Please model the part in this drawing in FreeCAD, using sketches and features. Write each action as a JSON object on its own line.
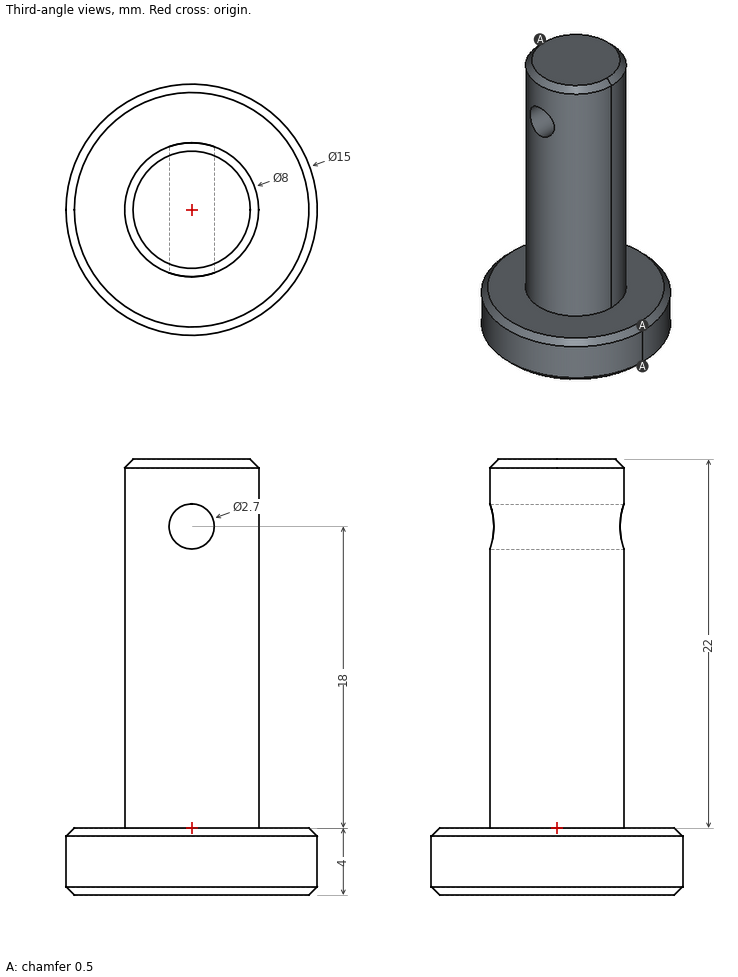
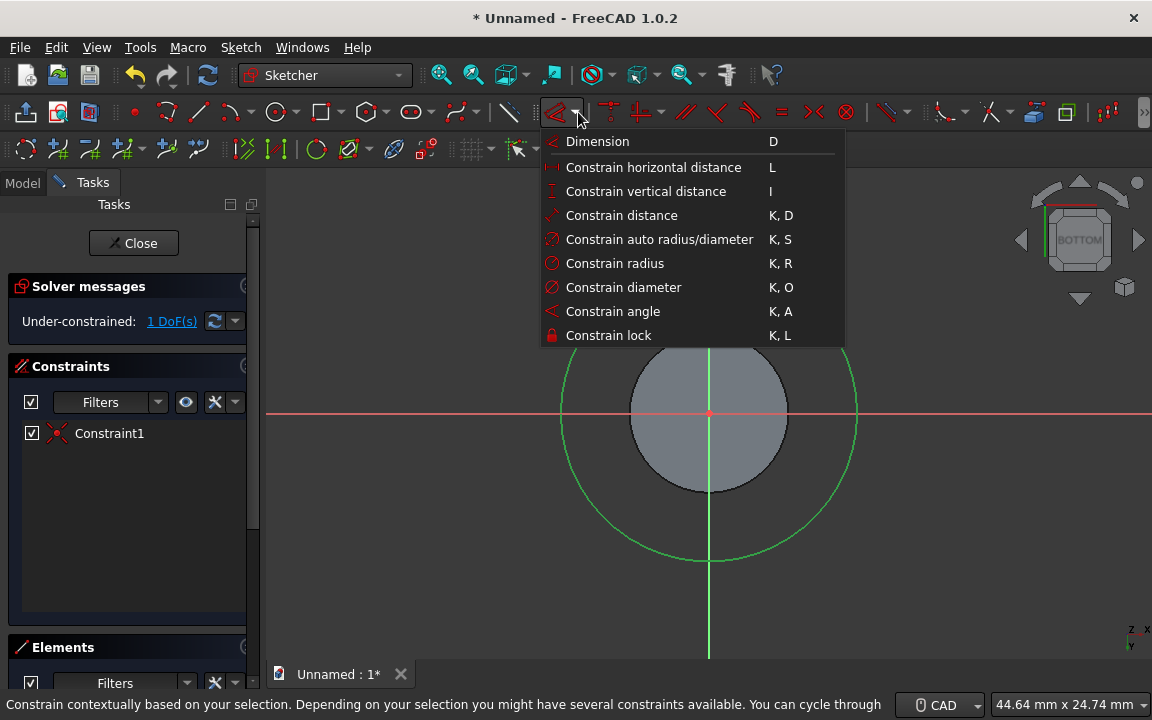
{"action": "left_click", "coordinate": [693, 287]}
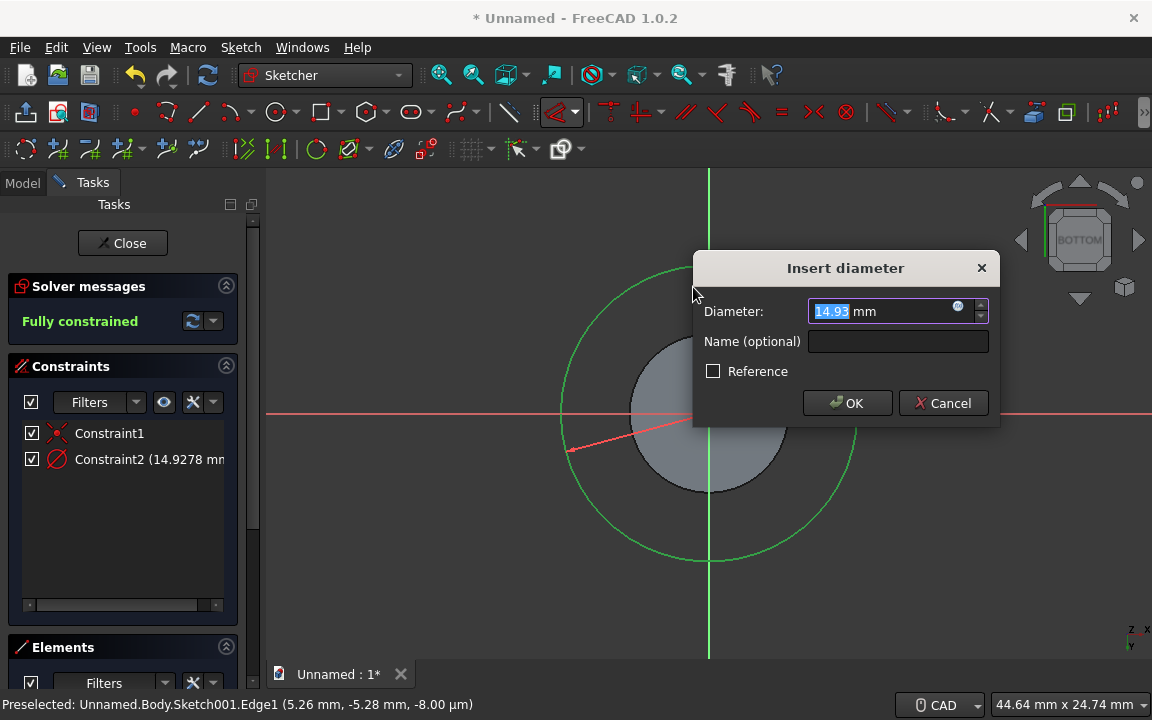
{"action": "type", "text": "15"}
{"action": "key", "text": "Return"}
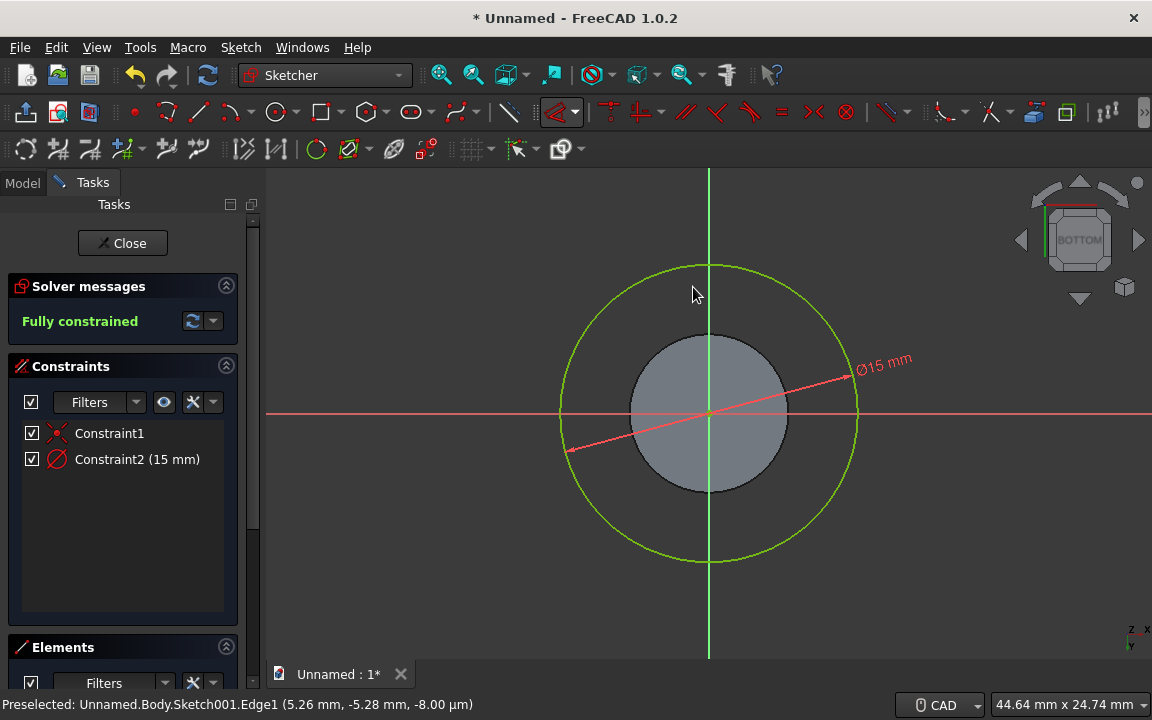
{"action": "left_click", "coordinate": [123, 243]}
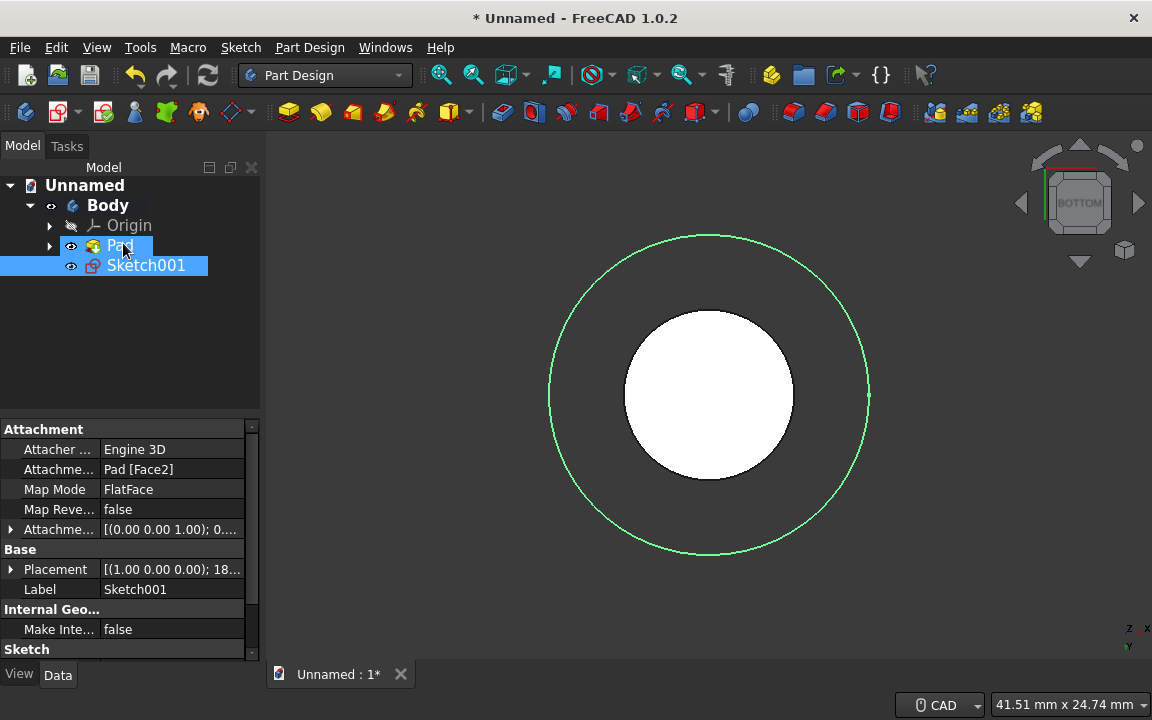
{"action": "left_click", "coordinate": [290, 112]}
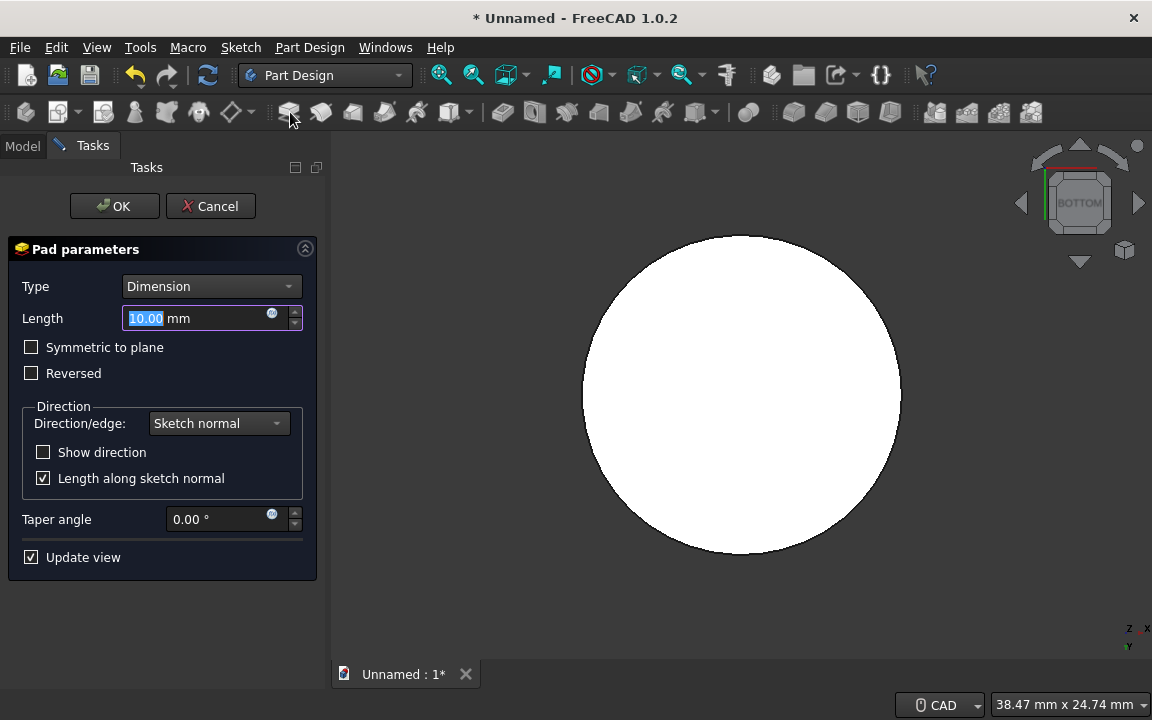
{"action": "type", "text": "4"}
{"action": "key", "text": "Tab"}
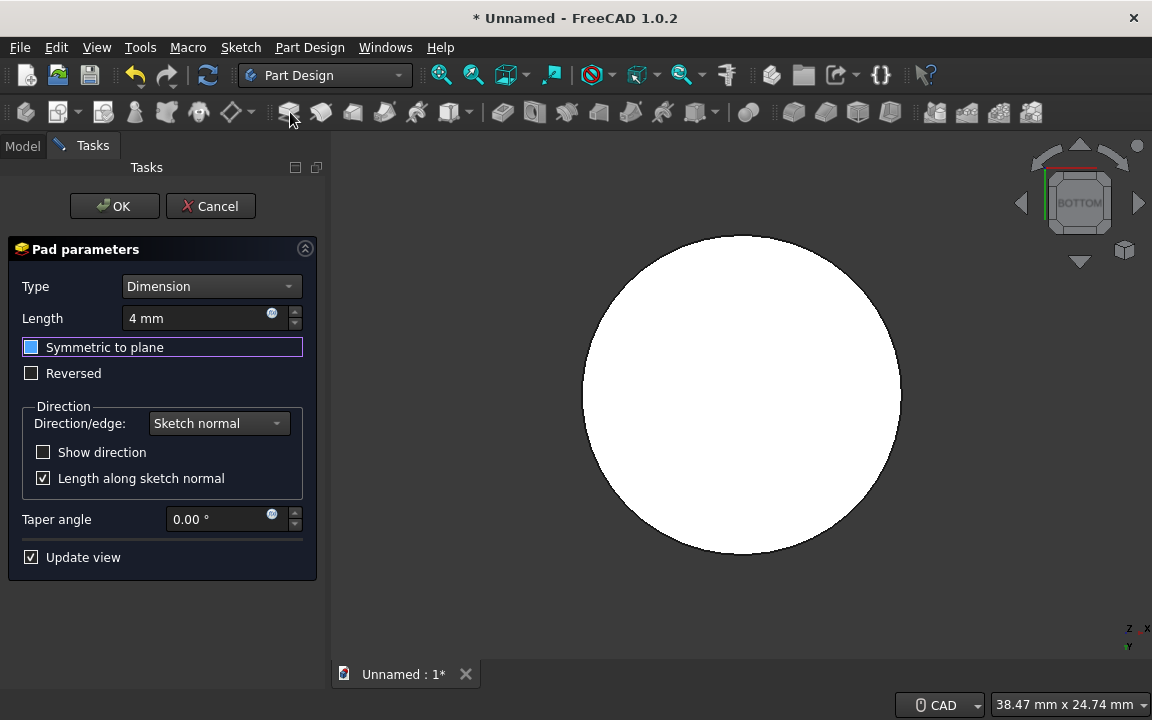
{"action": "left_click", "coordinate": [115, 206]}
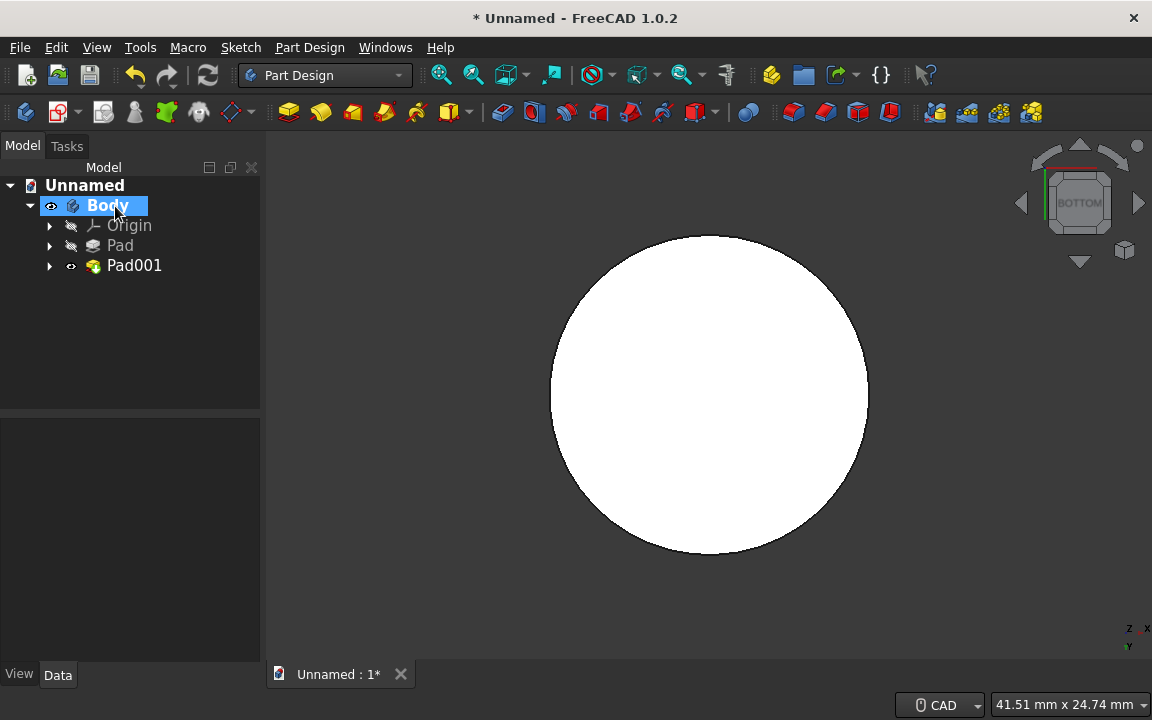
{"action": "left_click", "coordinate": [58, 112]}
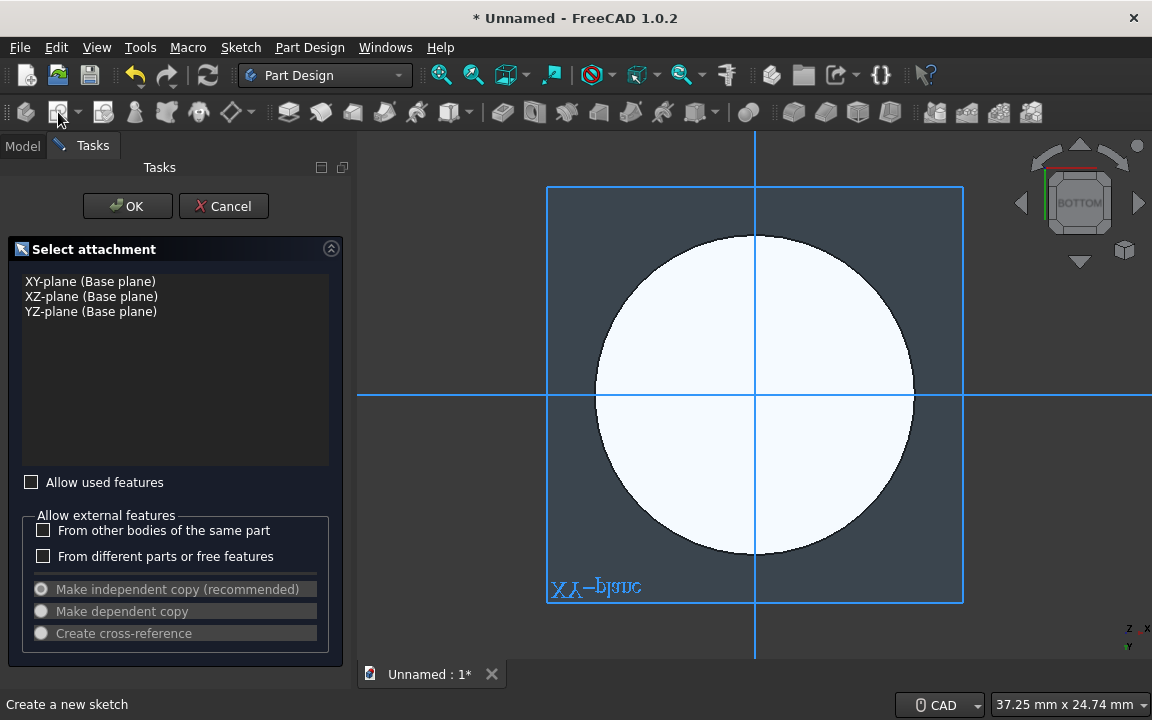
{"action": "left_click", "coordinate": [82, 296]}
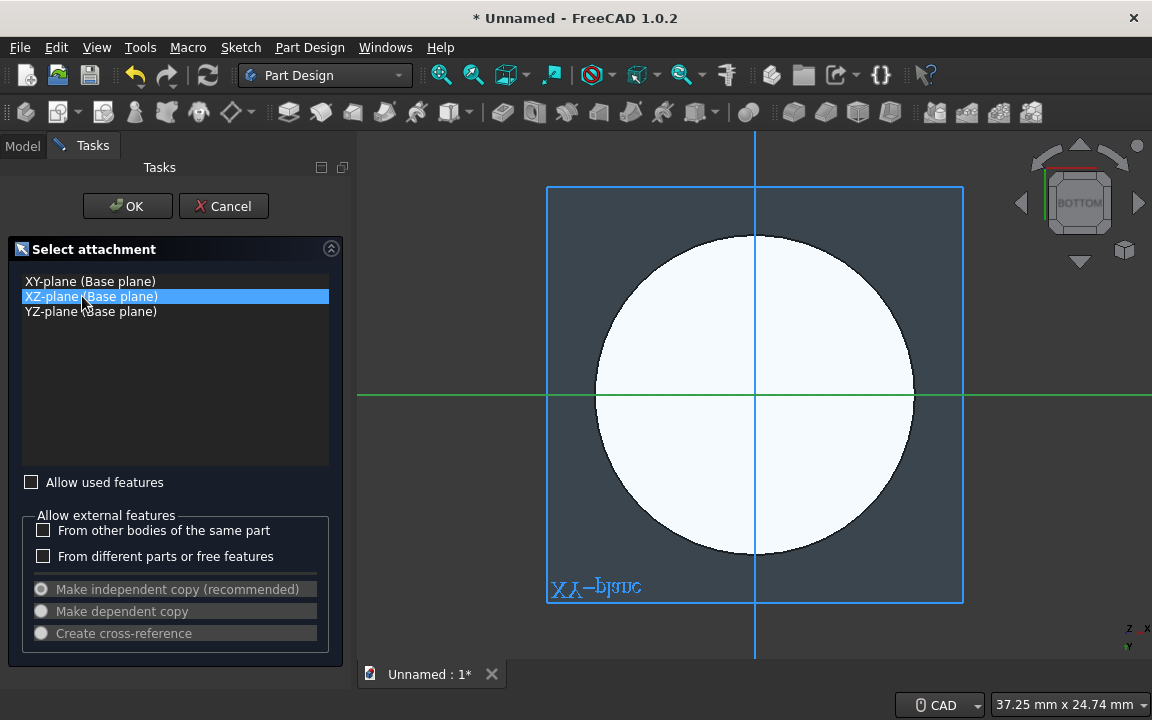
{"action": "left_click", "coordinate": [128, 206]}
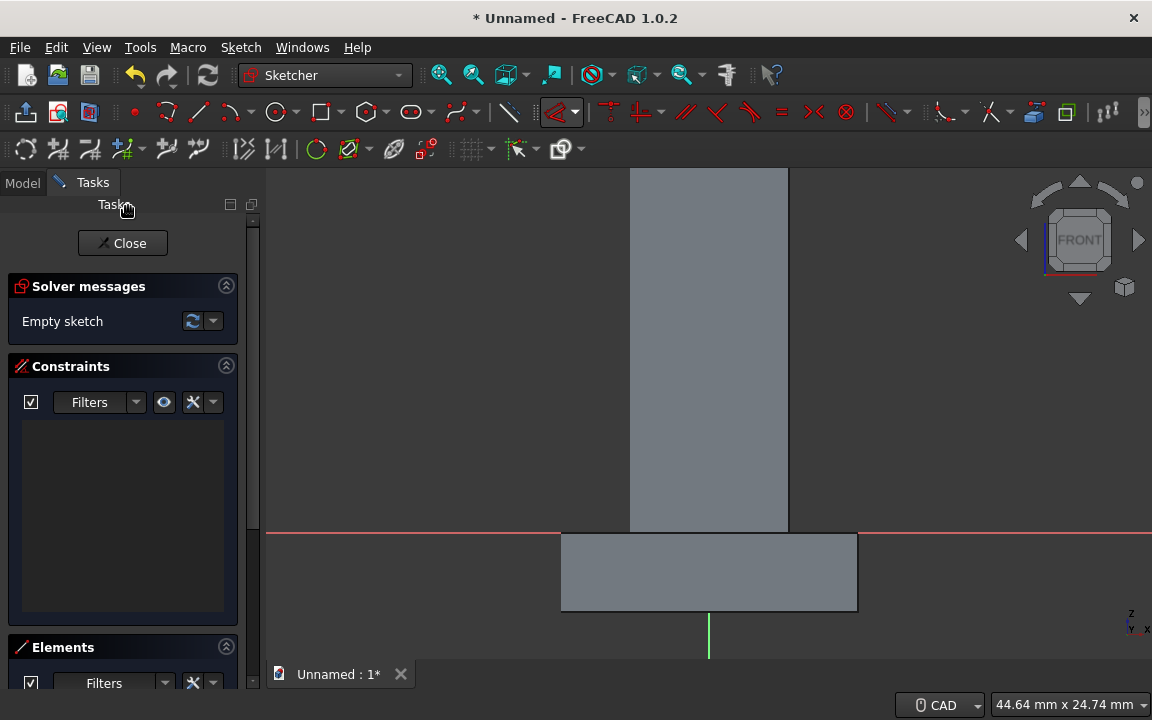
{"action": "left_click", "coordinate": [90, 112]}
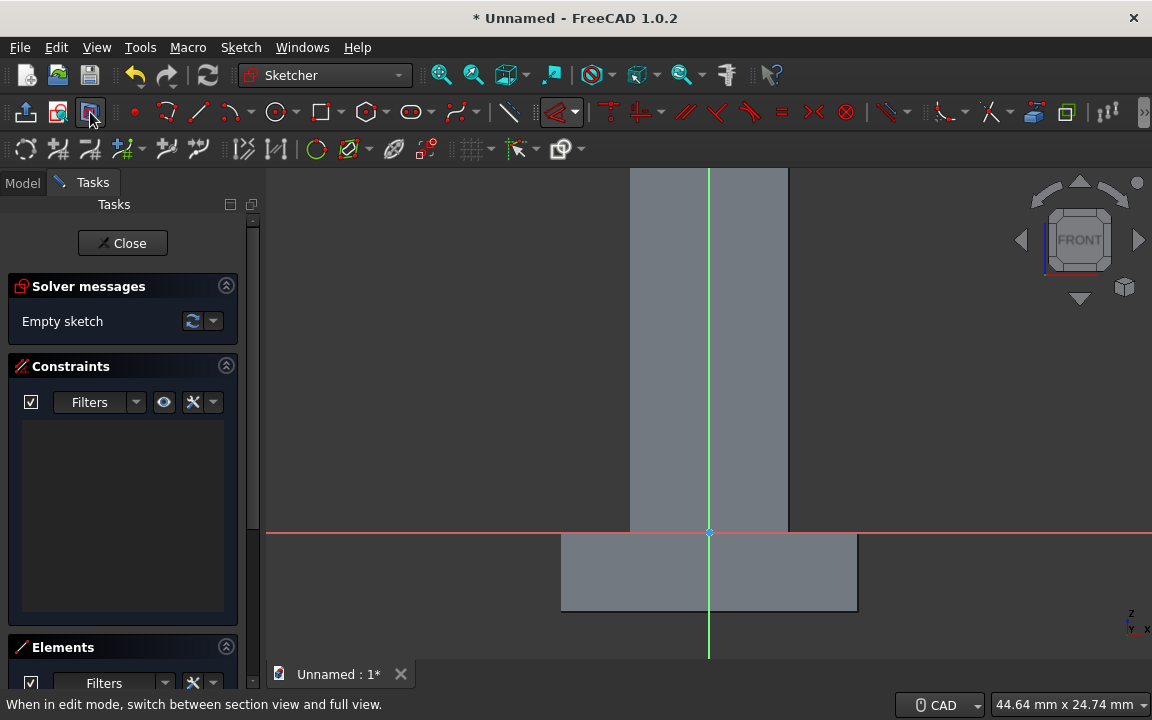
{"action": "scroll", "coordinate": [640, 414], "scroll_direction": "down", "scroll_amount": 5}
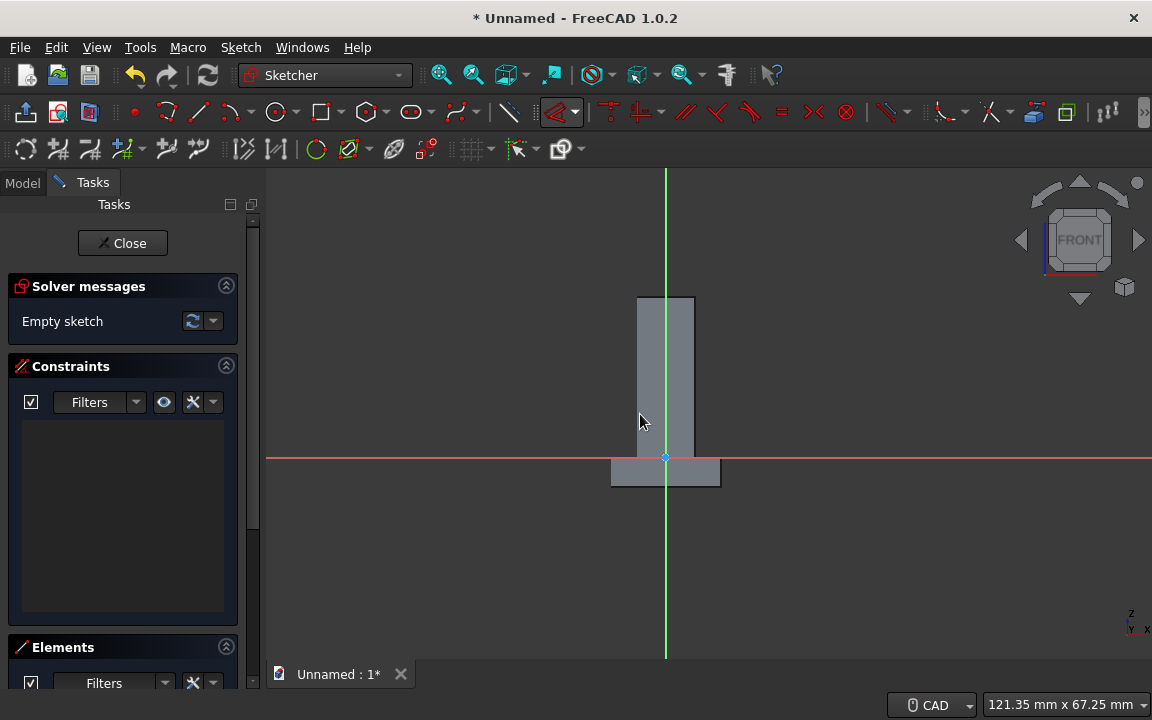
{"action": "scroll", "coordinate": [667, 321], "scroll_direction": "up", "scroll_amount": 14}